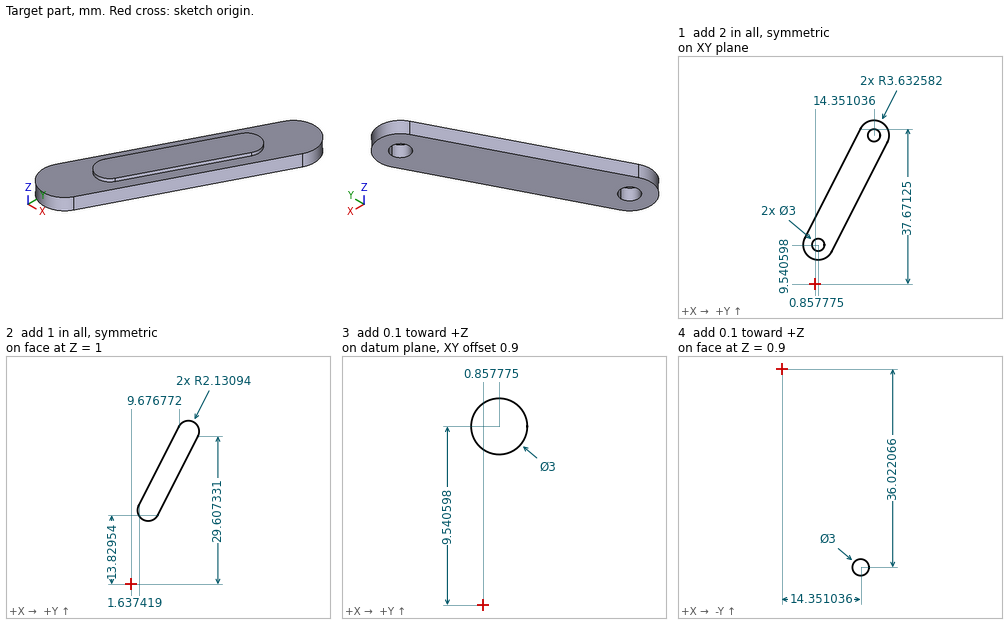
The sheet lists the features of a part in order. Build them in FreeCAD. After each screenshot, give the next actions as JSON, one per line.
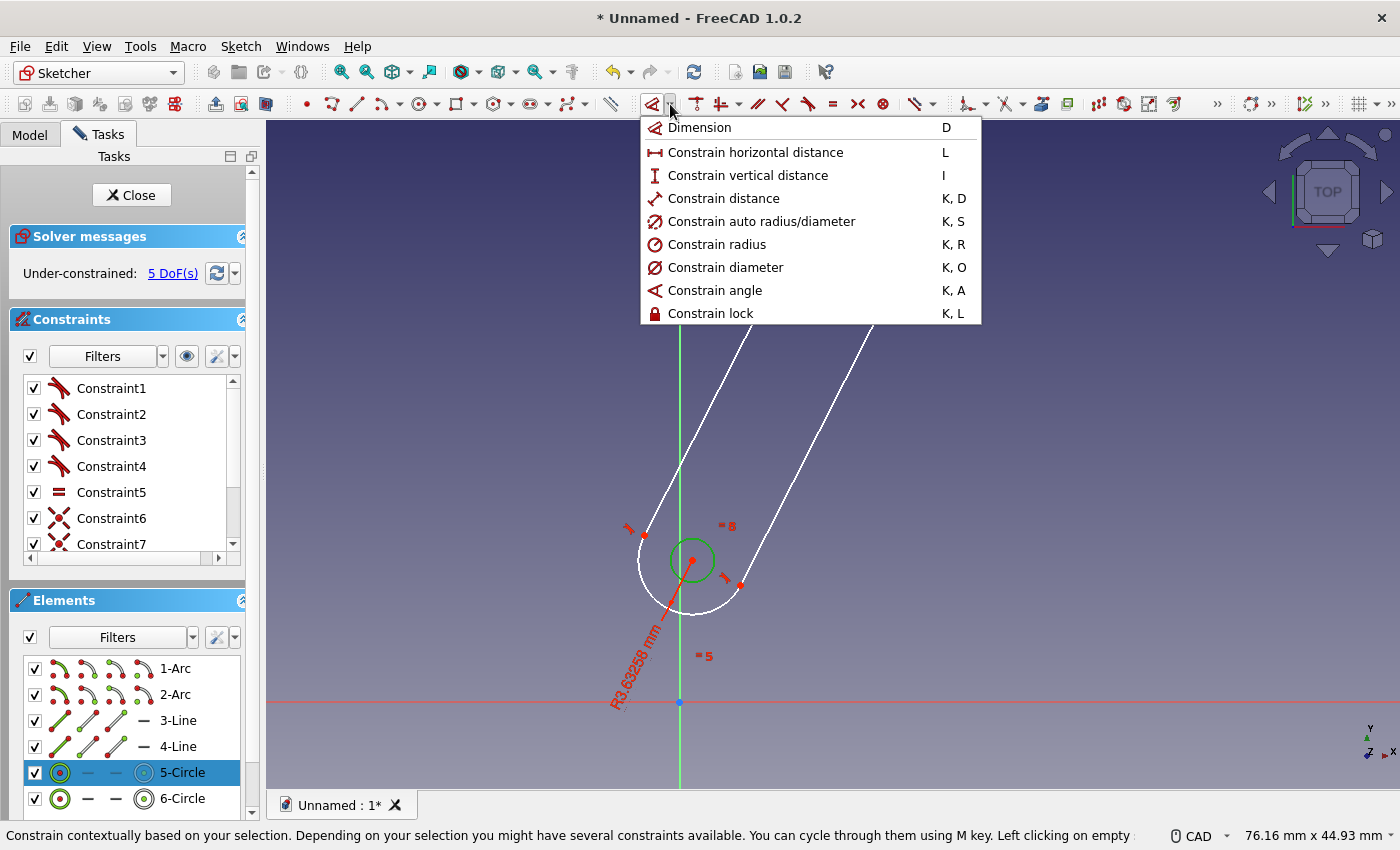
{"action": "left_click", "coordinate": [811, 268]}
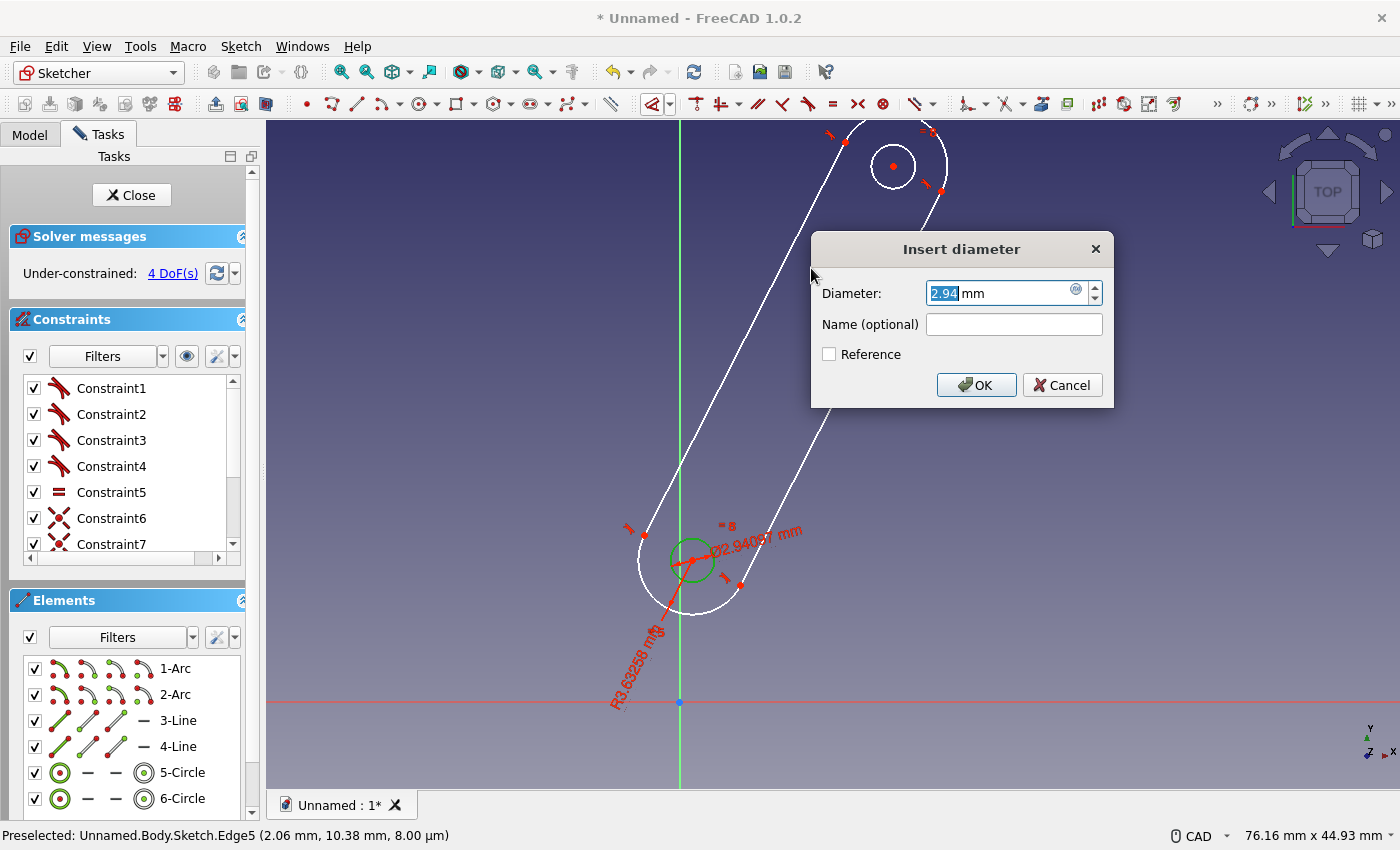
{"action": "type", "text": "3"}
{"action": "key", "text": "Return"}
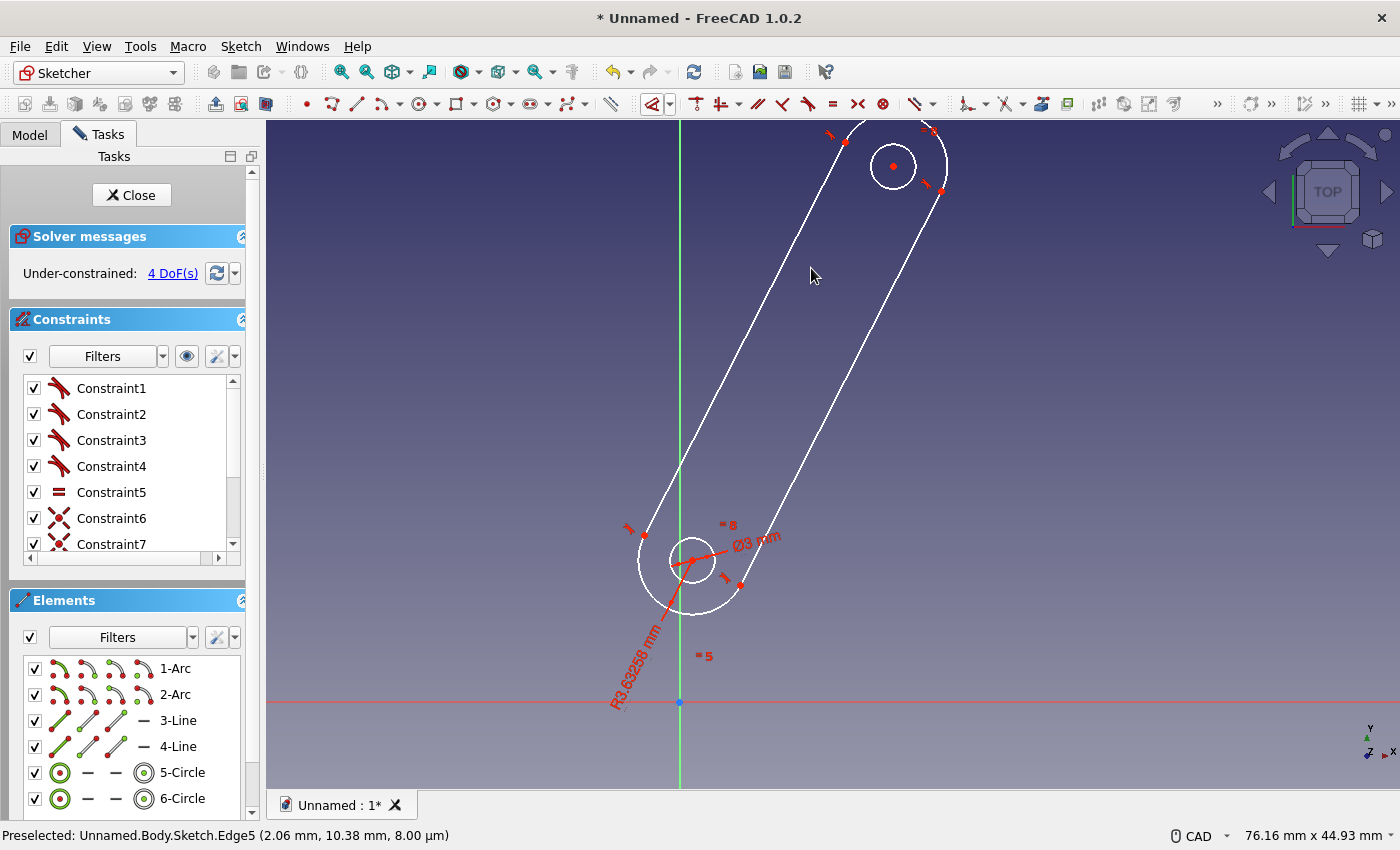
{"action": "scroll", "coordinate": [693, 560], "scroll_direction": "up", "scroll_amount": 6}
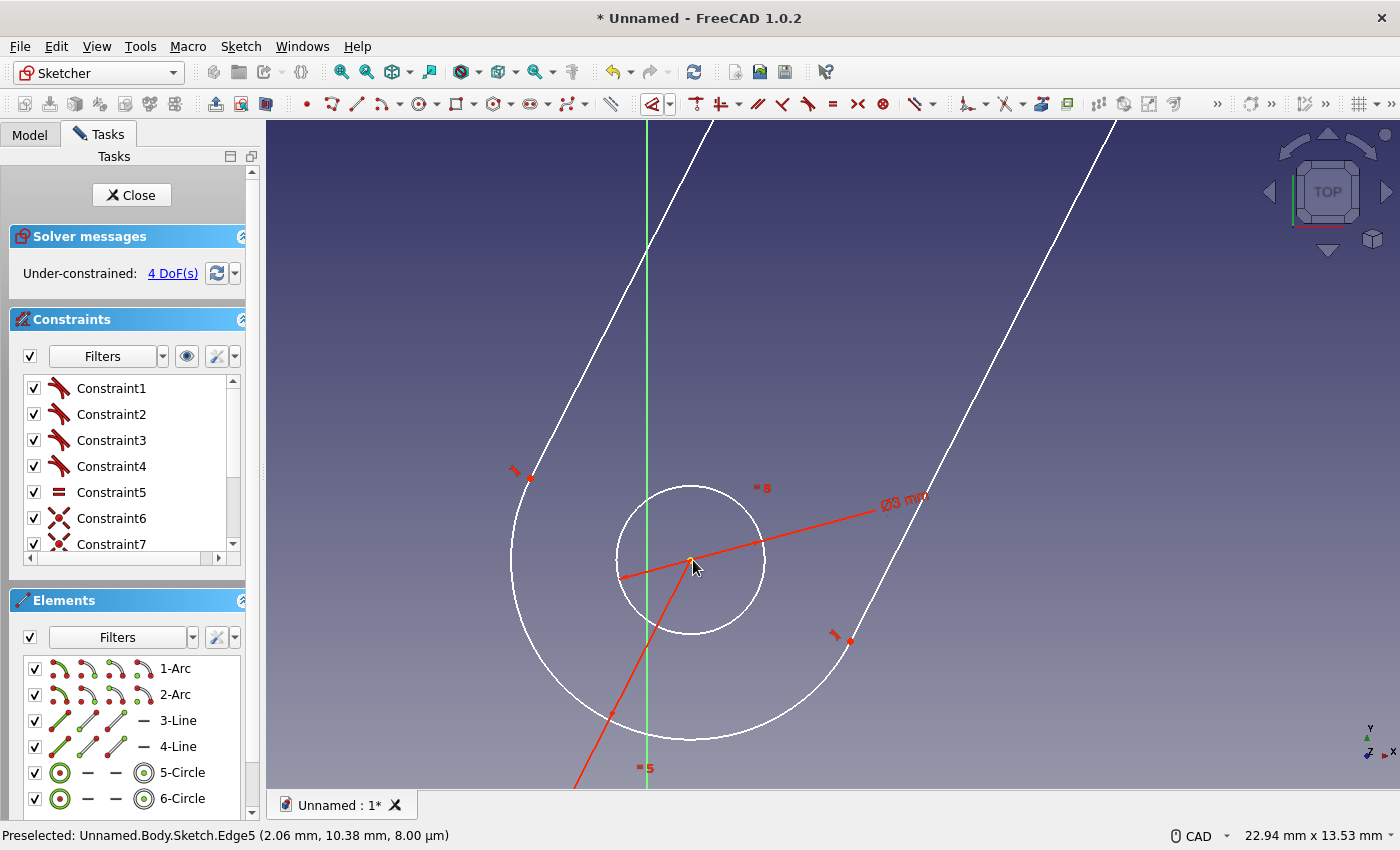
{"action": "left_click", "coordinate": [691, 560]}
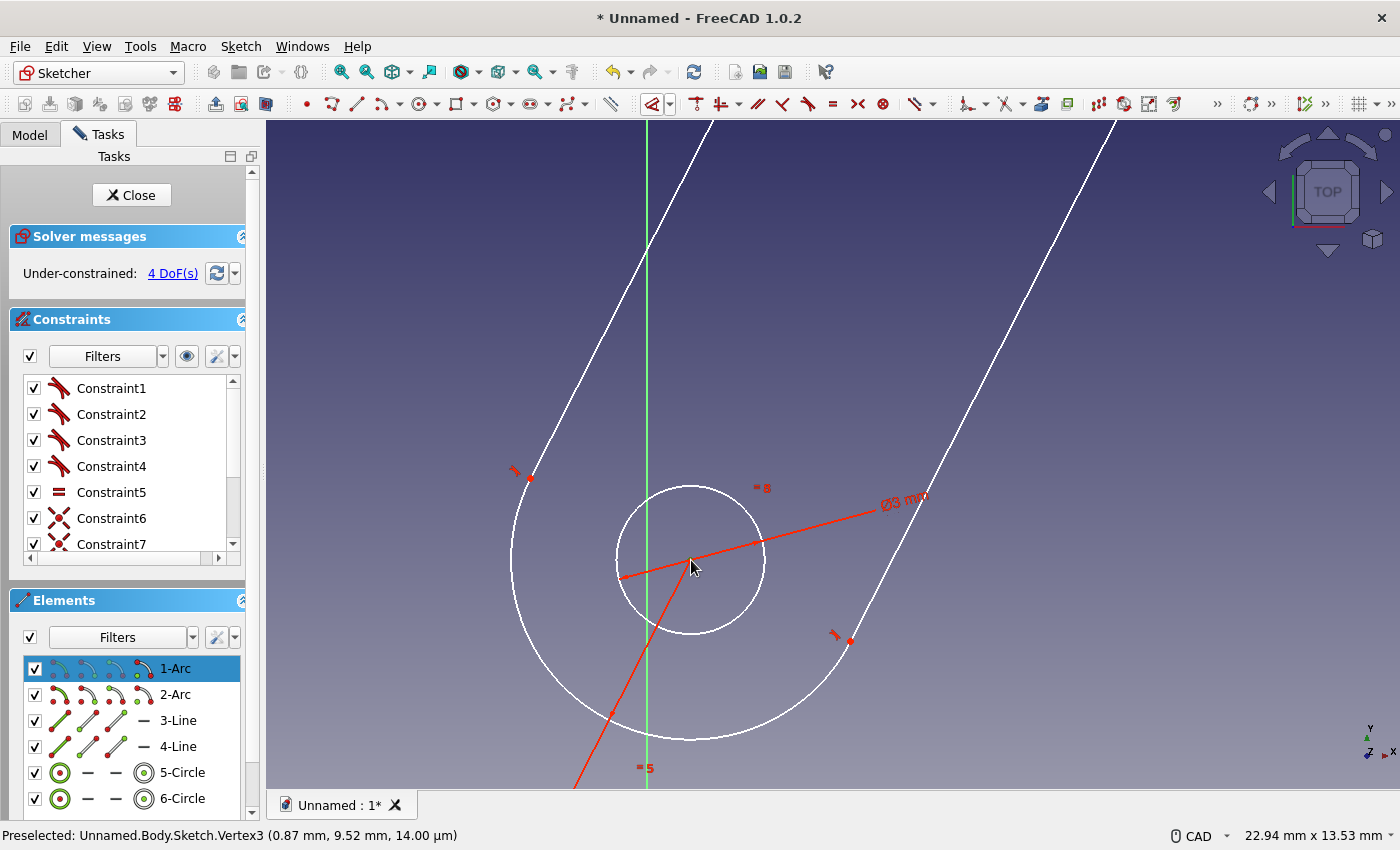
{"action": "key", "text": "l"}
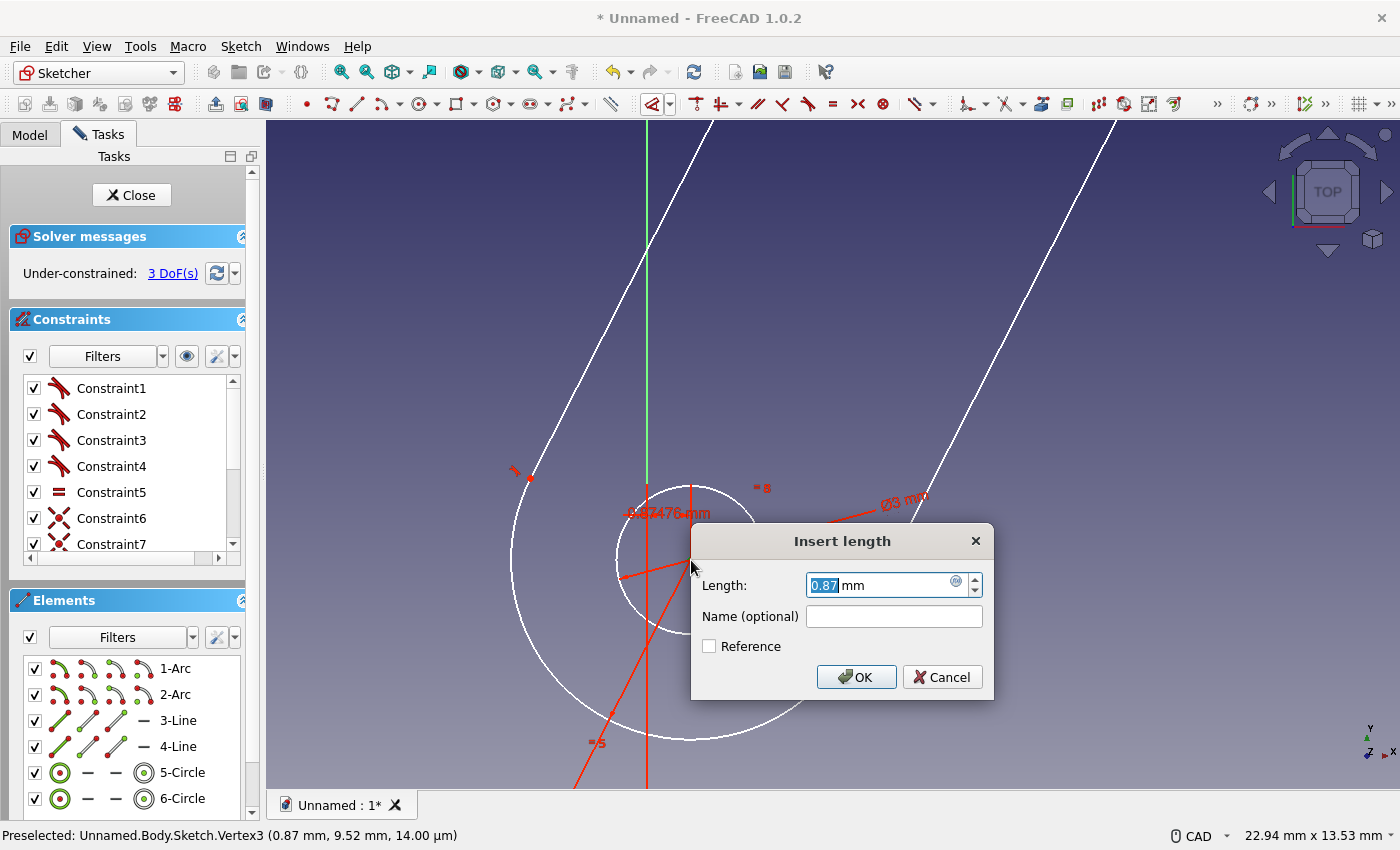
{"action": "type", "text": "0.857775"}
{"action": "key", "text": "Return"}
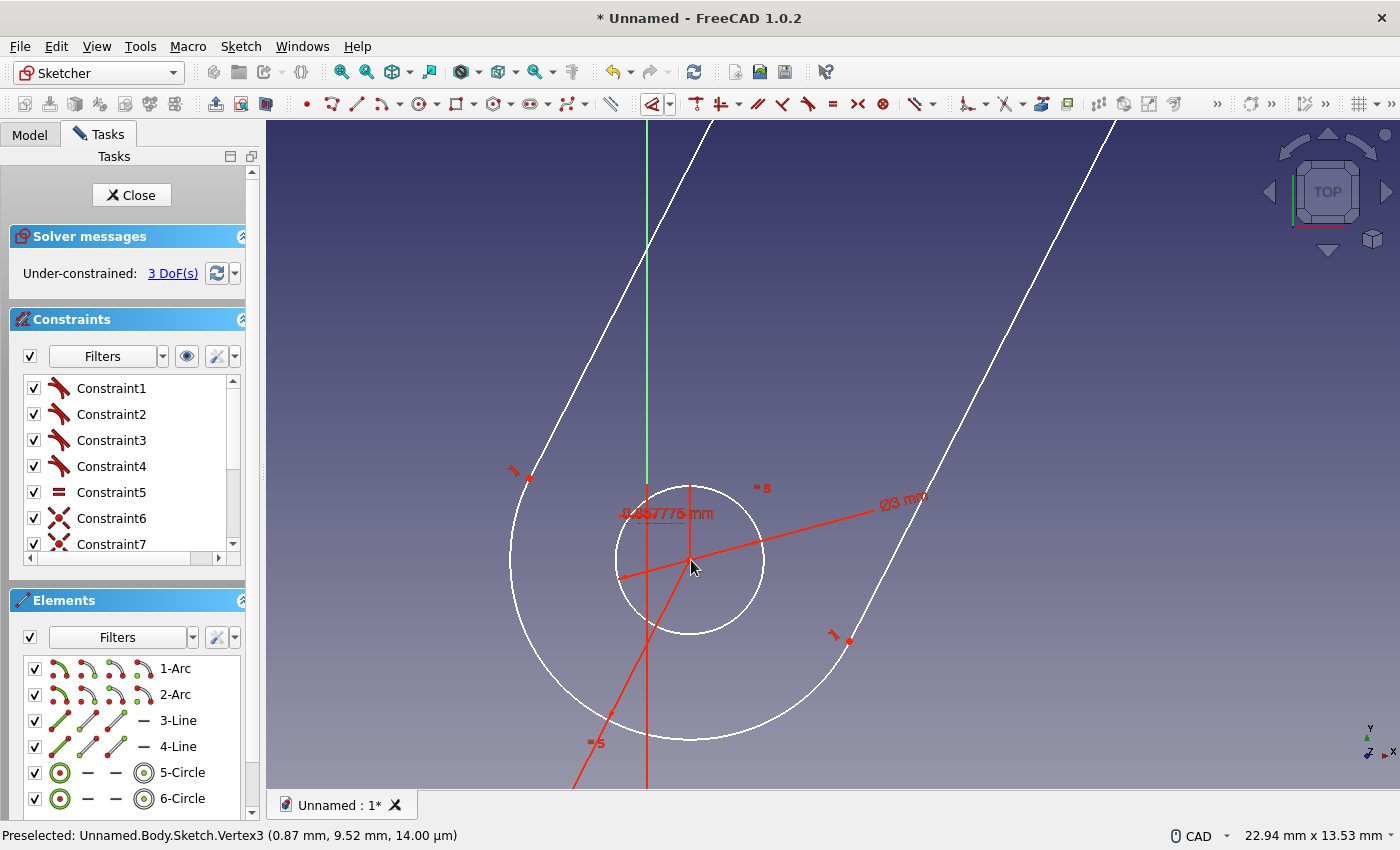
{"action": "scroll", "coordinate": [699, 554], "scroll_direction": "down", "scroll_amount": 8}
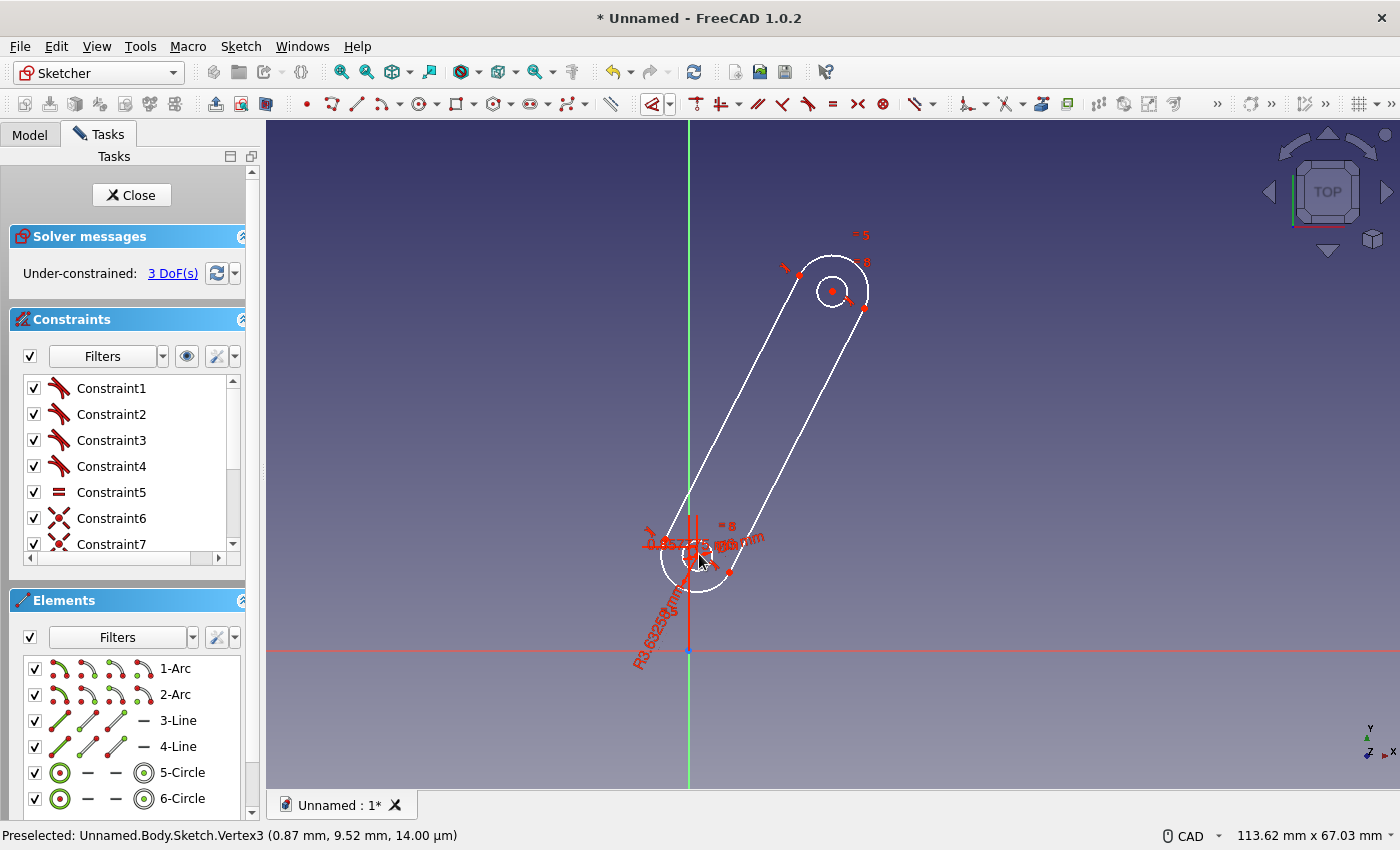
{"action": "left_click", "coordinate": [697, 556]}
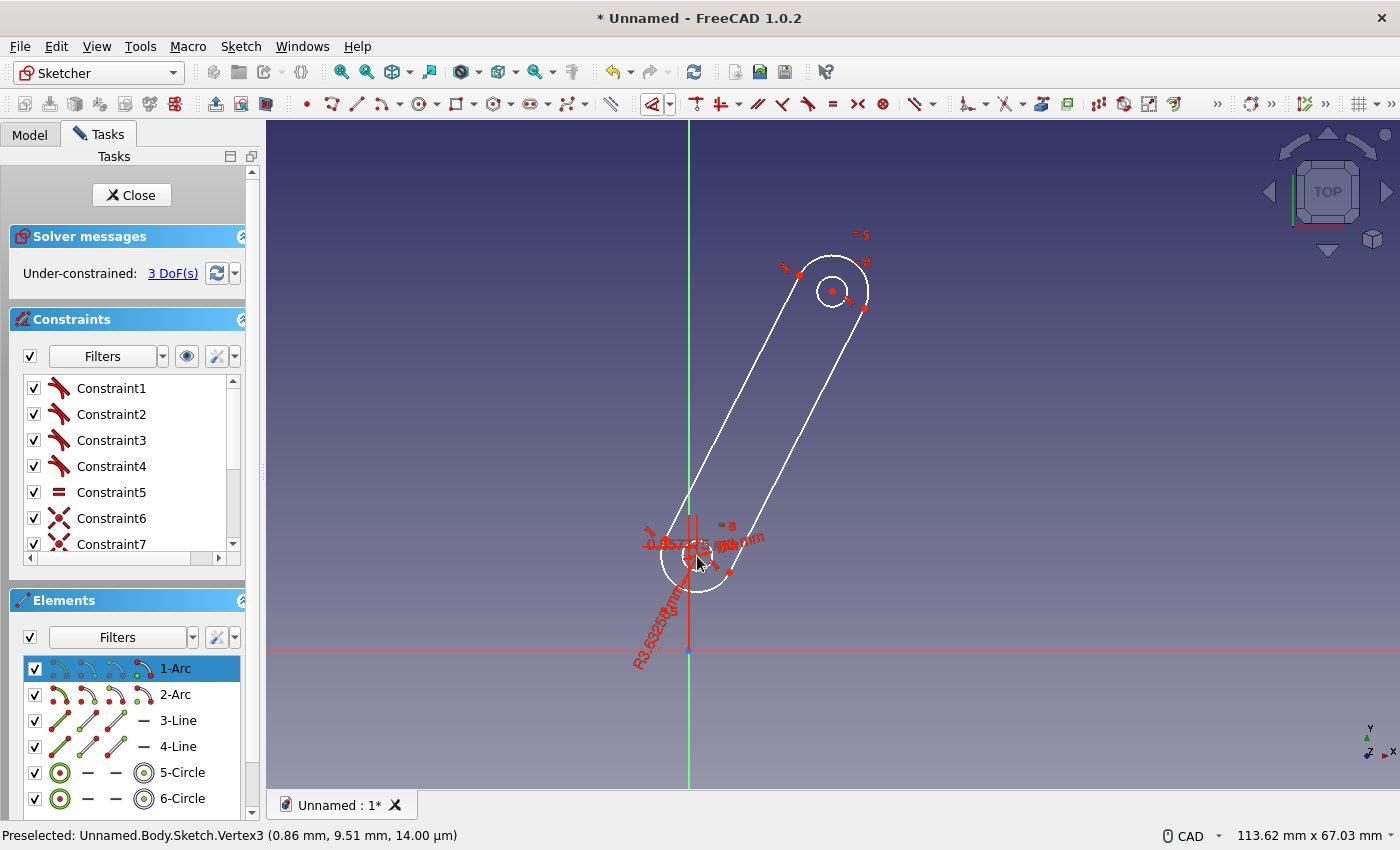
{"action": "key", "text": "i"}